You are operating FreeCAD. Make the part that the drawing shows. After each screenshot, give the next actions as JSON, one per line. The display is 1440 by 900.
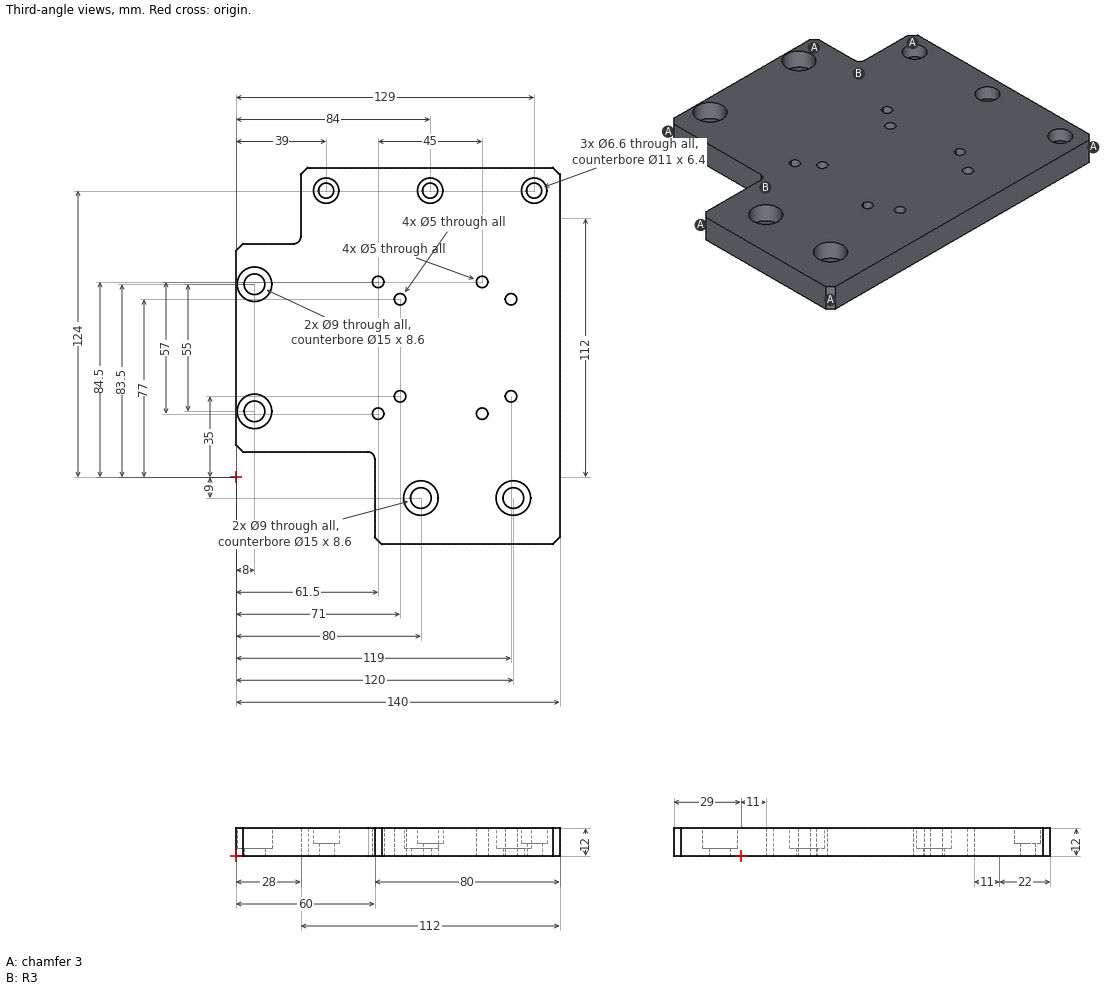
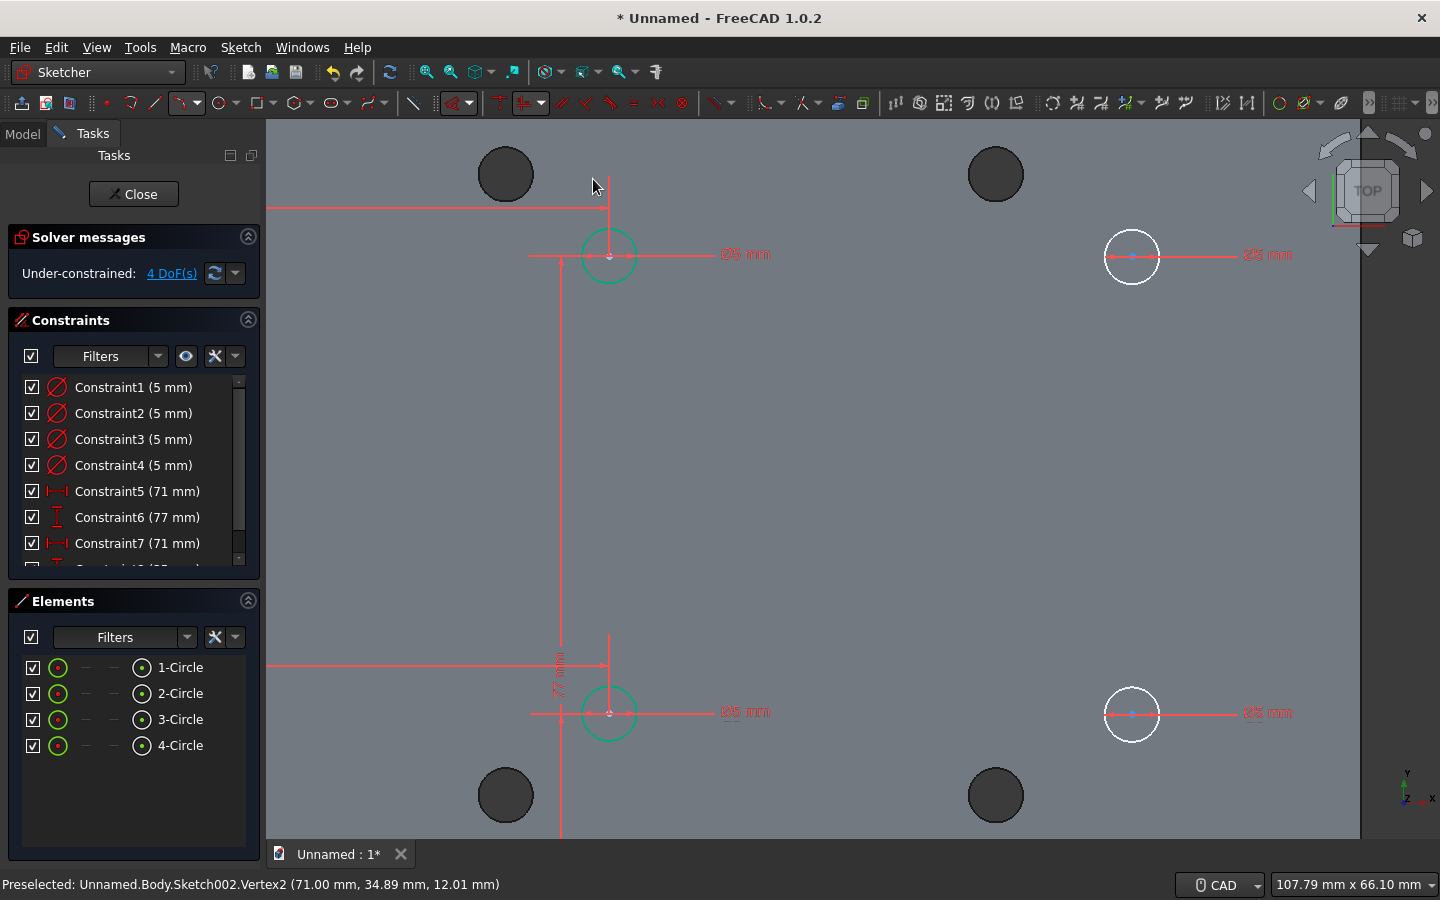
{"action": "left_click", "coordinate": [1132, 715]}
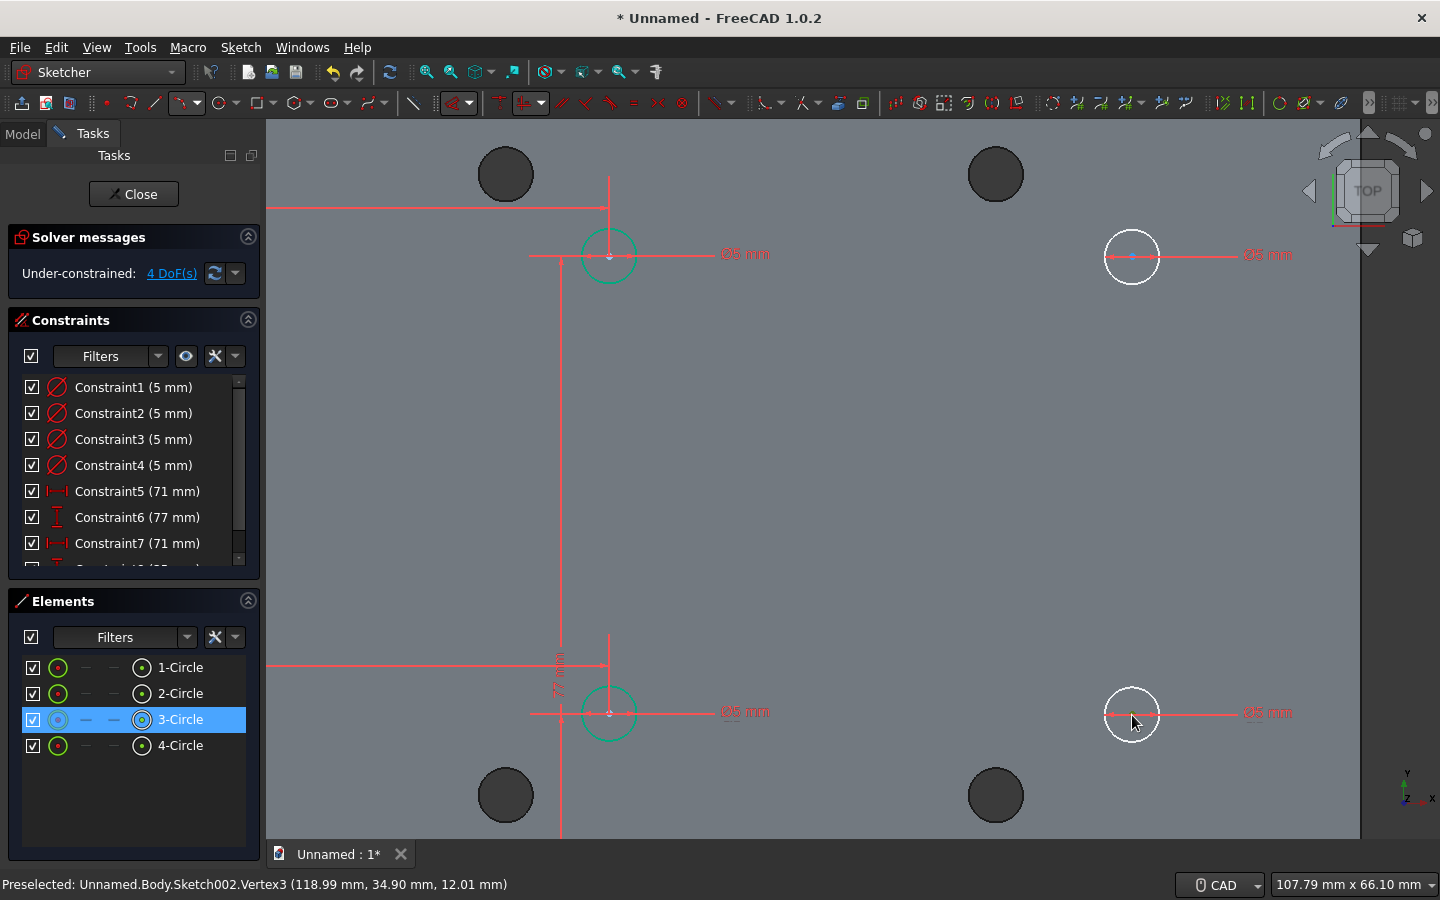
{"action": "left_click", "coordinate": [472, 104]}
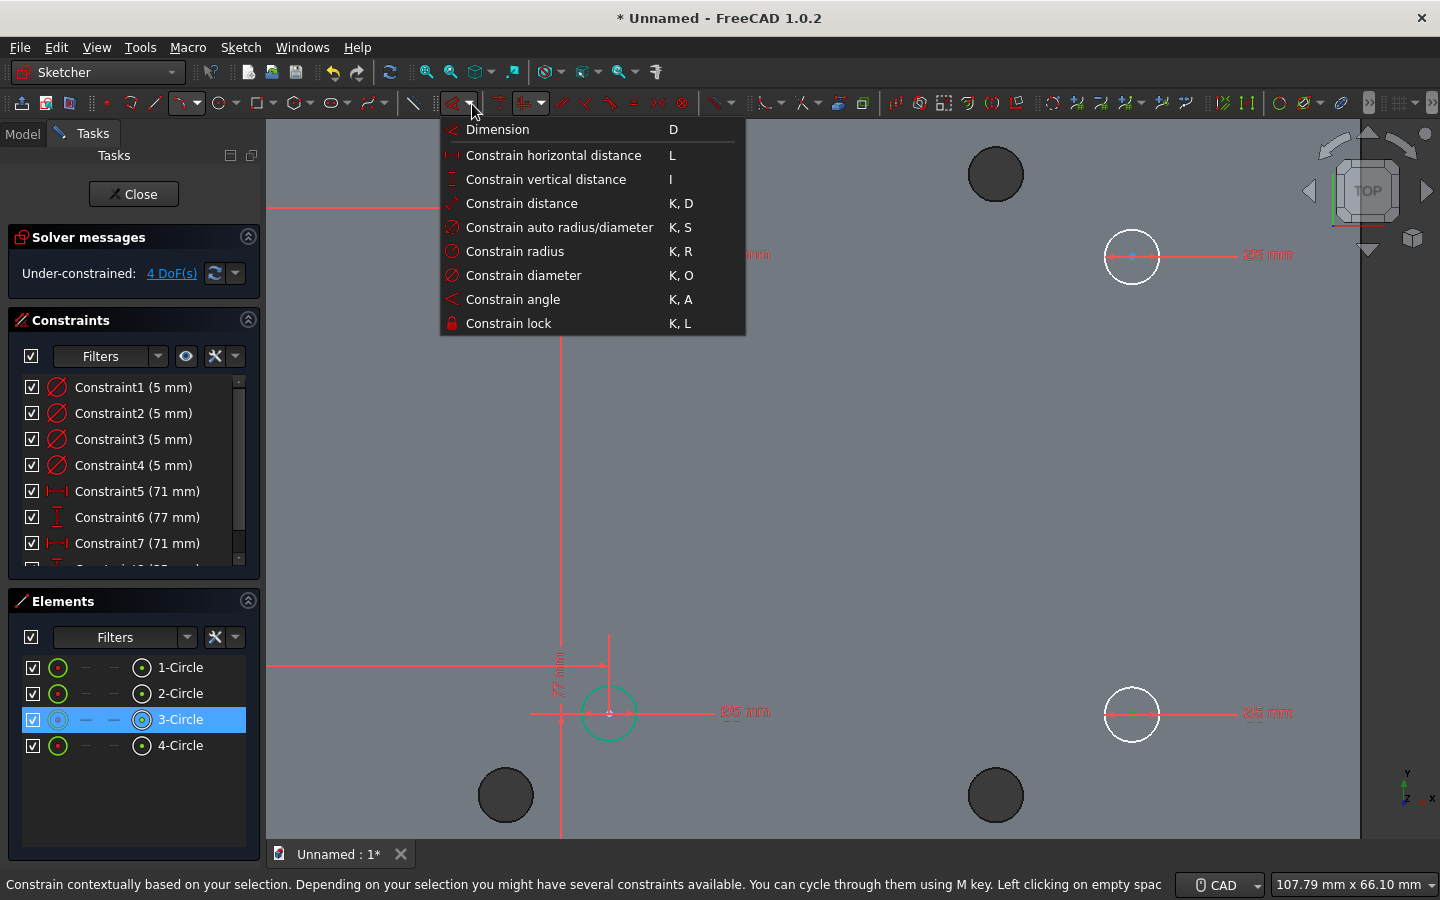
{"action": "left_click", "coordinate": [593, 179]}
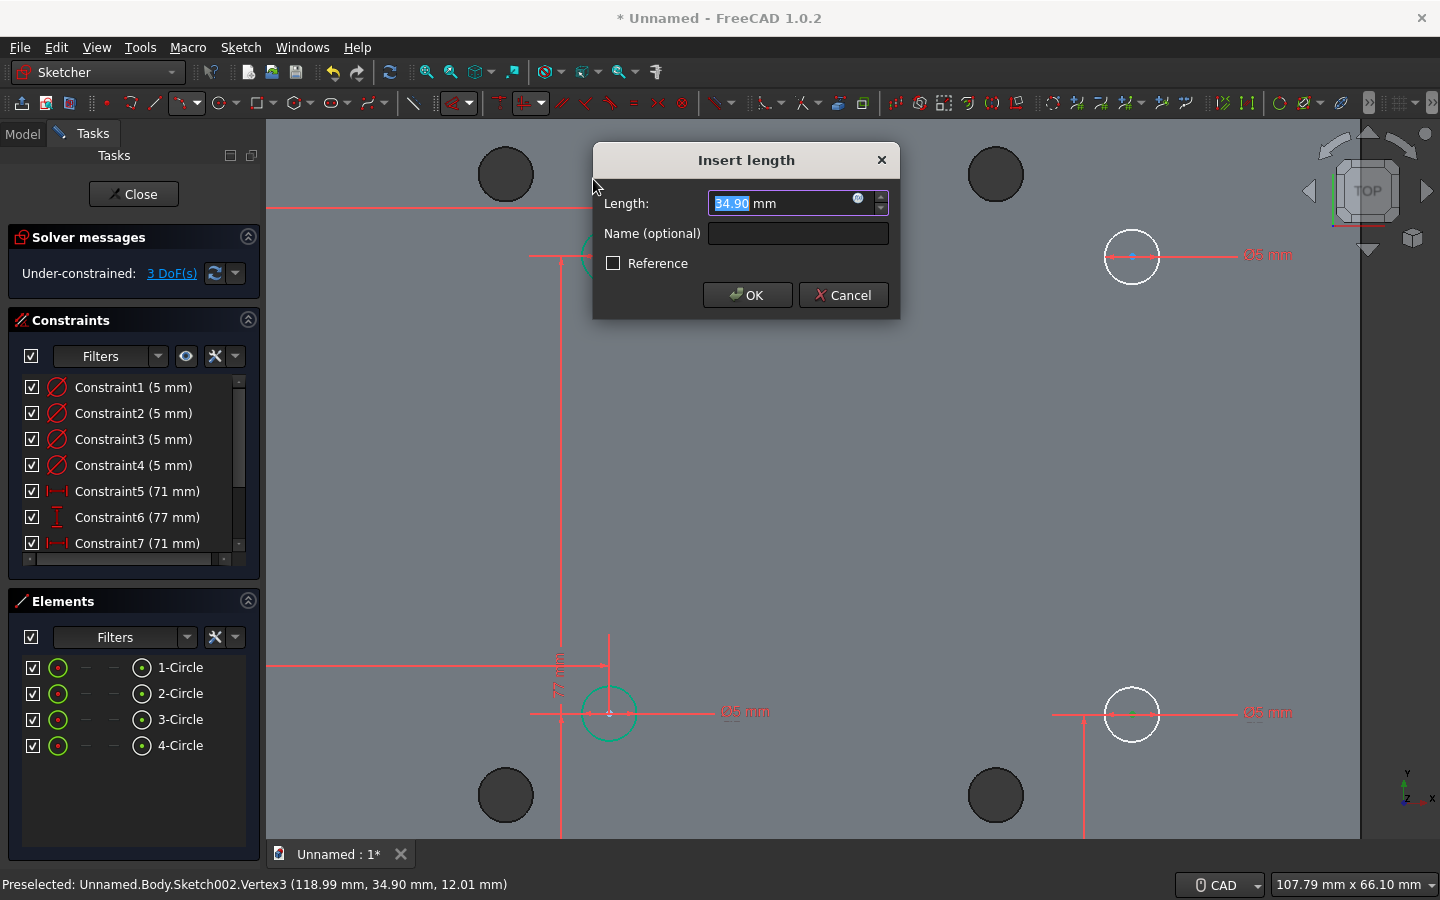
{"action": "type", "text": "35"}
{"action": "key", "text": "Return"}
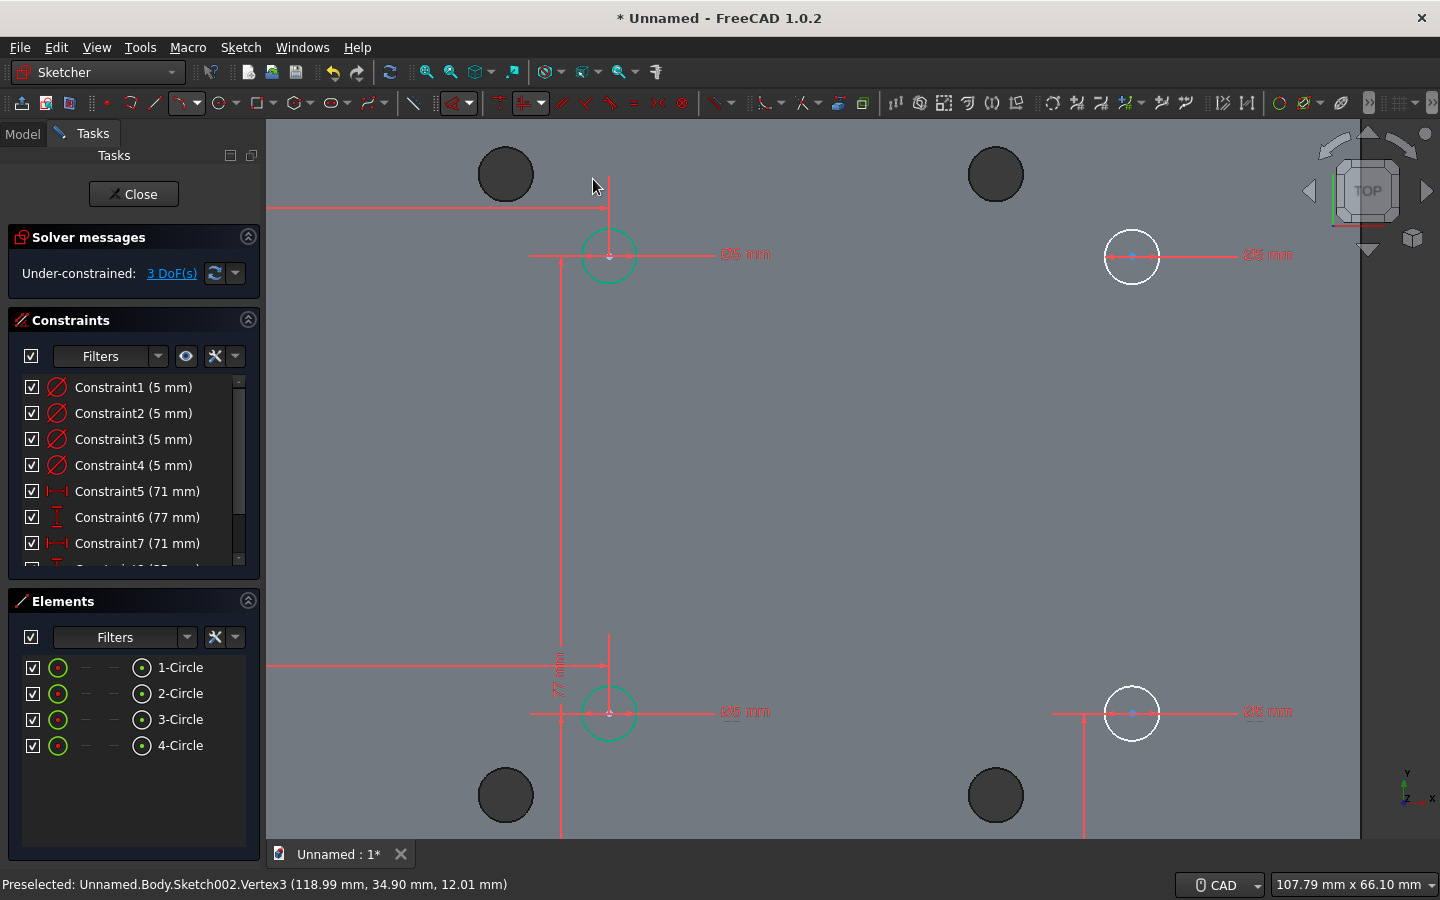
{"action": "left_click", "coordinate": [1132, 257]}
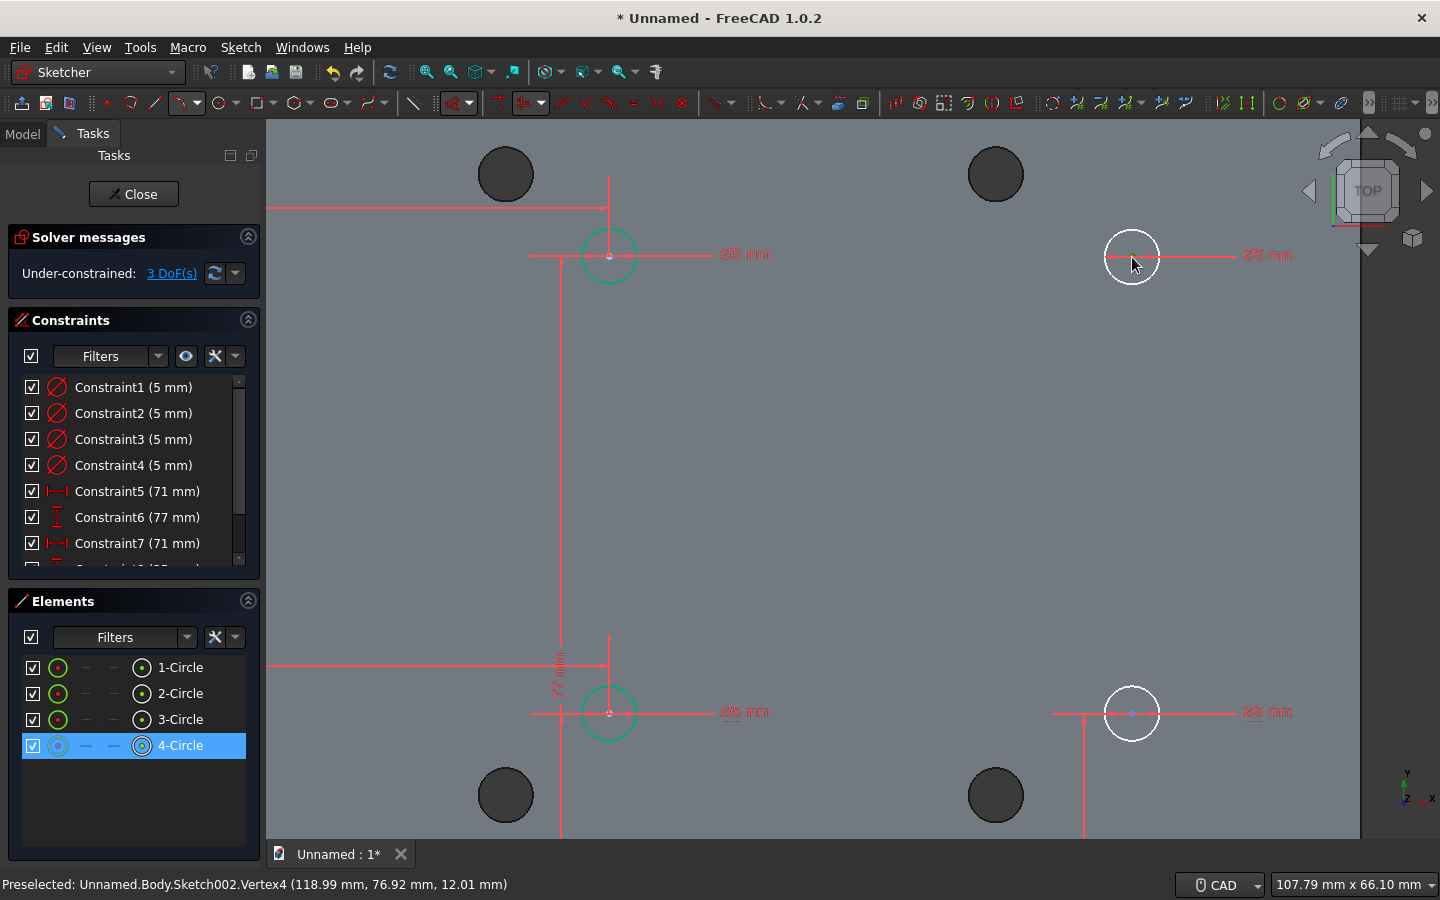
{"action": "key", "text": "i"}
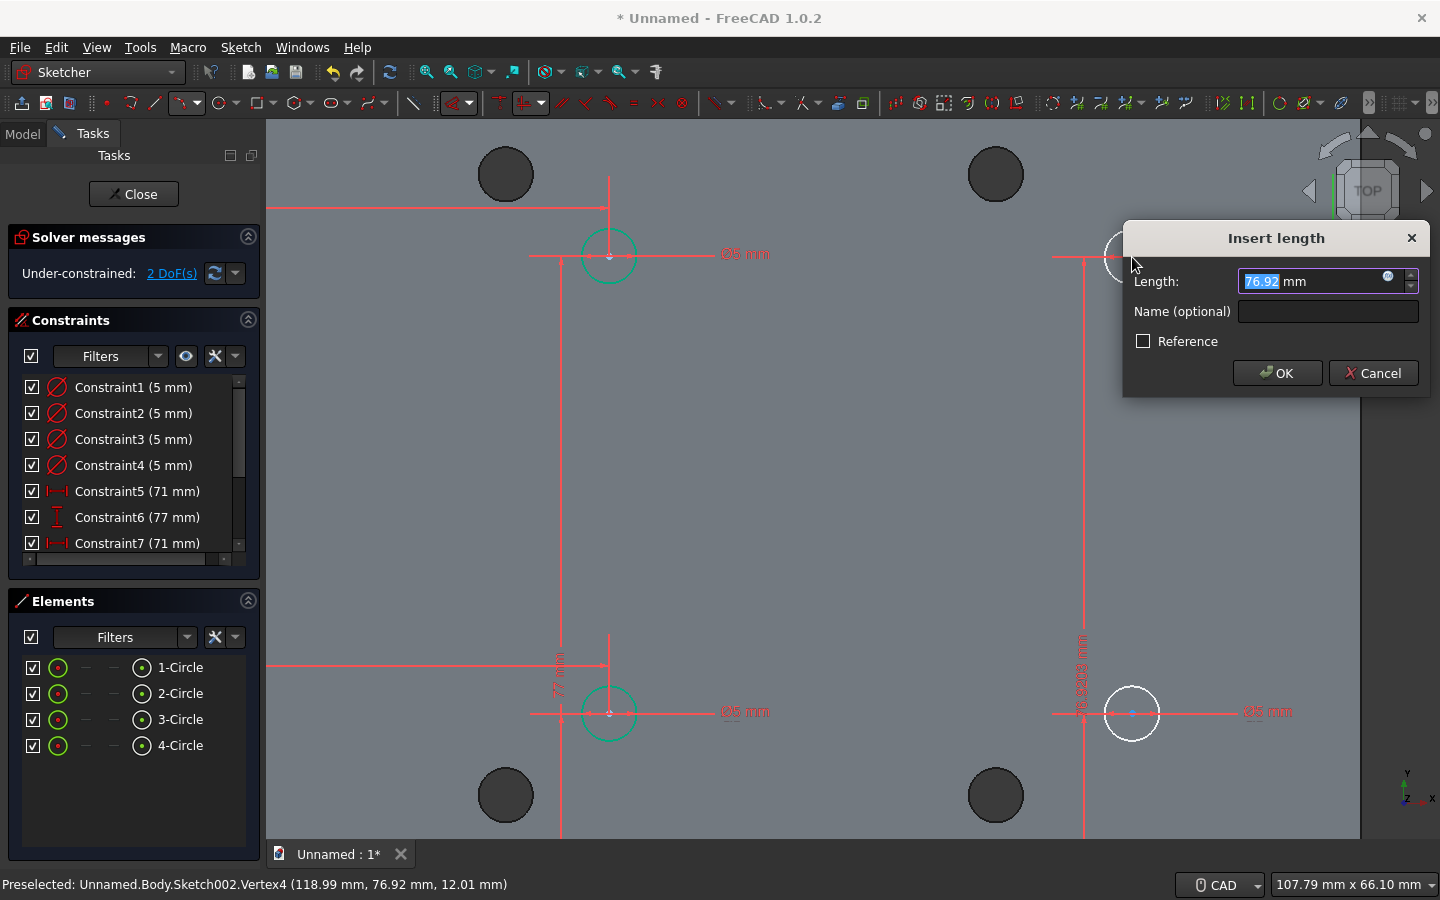
{"action": "type", "text": "77"}
{"action": "key", "text": "Return"}